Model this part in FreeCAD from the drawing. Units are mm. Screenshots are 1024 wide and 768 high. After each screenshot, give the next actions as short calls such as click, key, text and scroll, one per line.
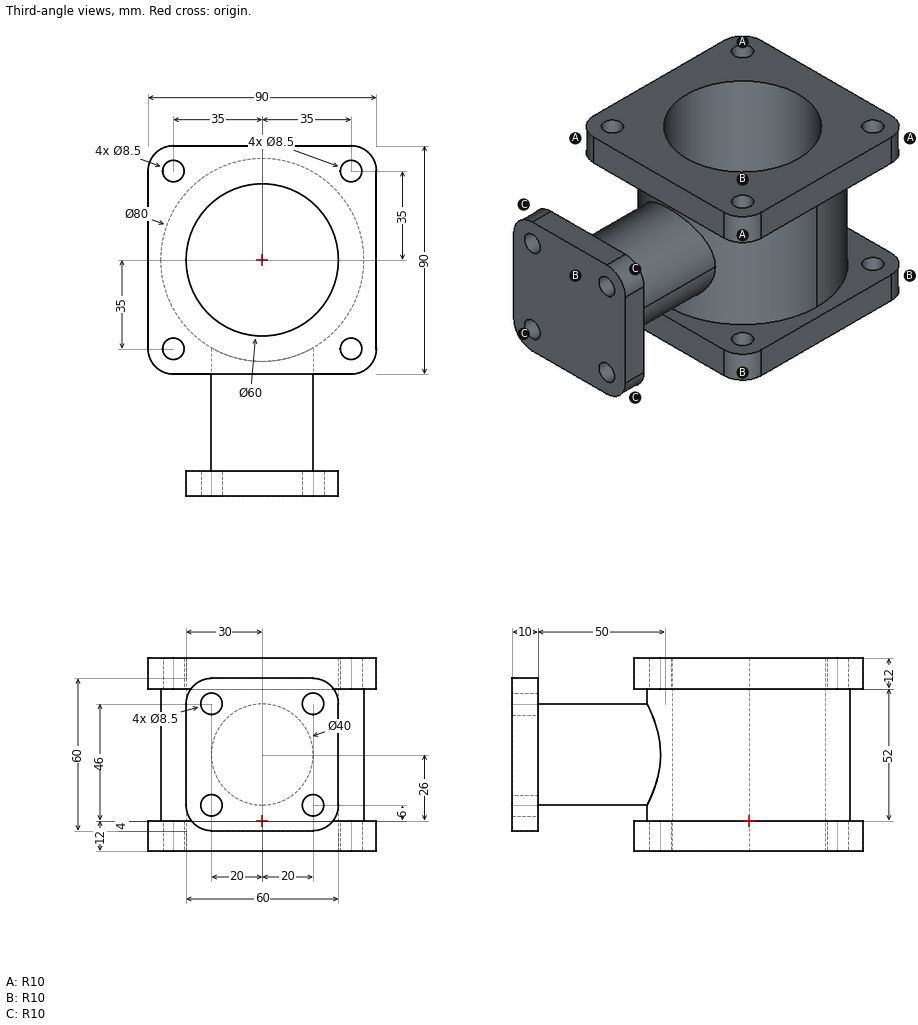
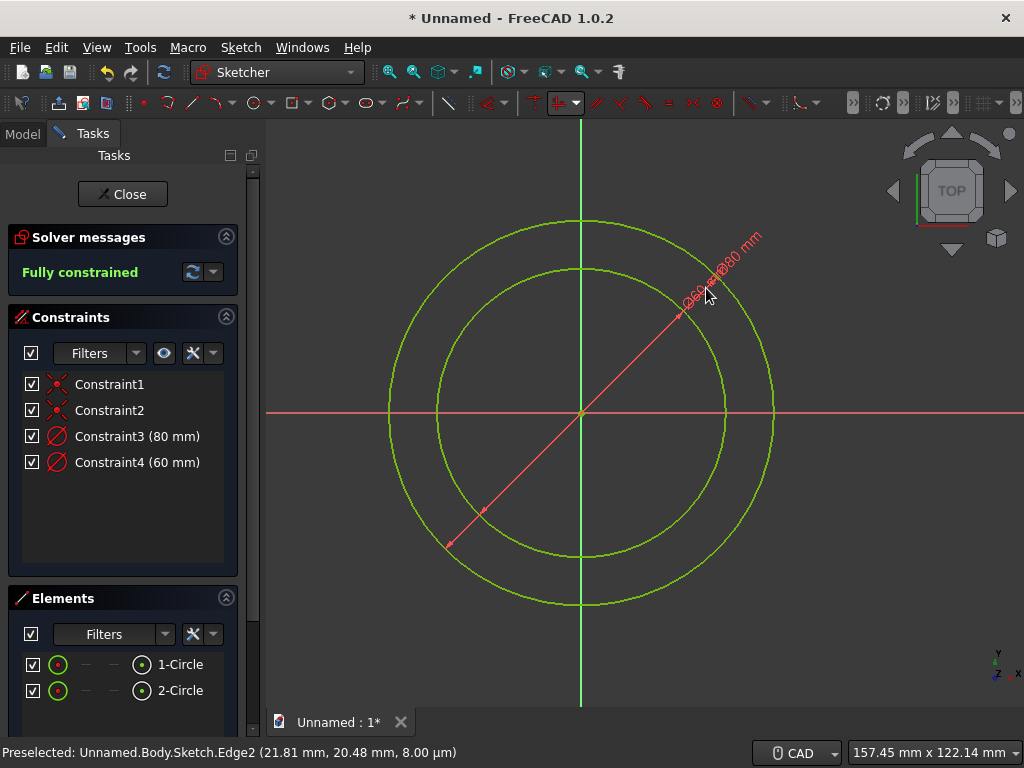
click(123, 194)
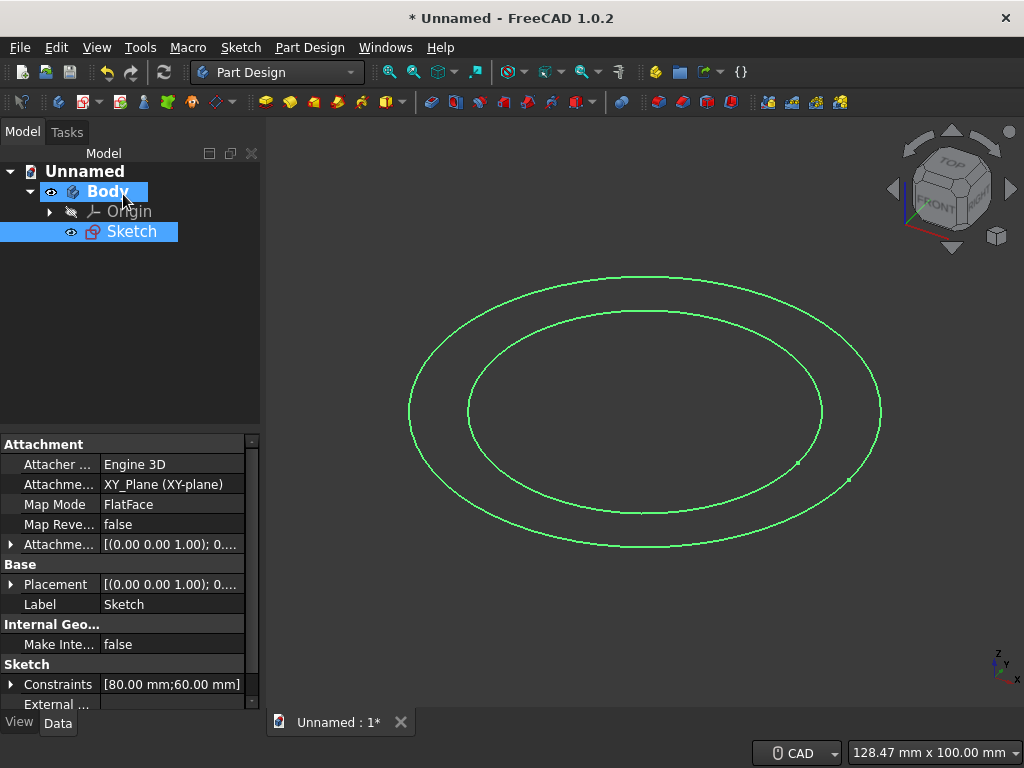
click(266, 102)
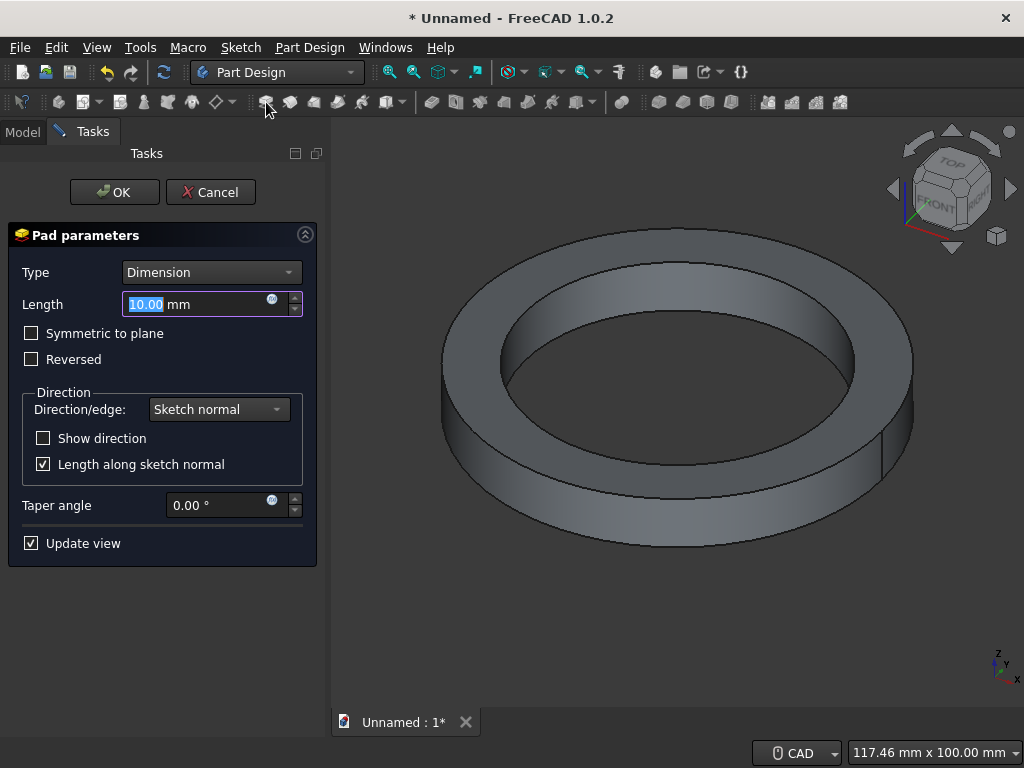
text(52)
key(Tab)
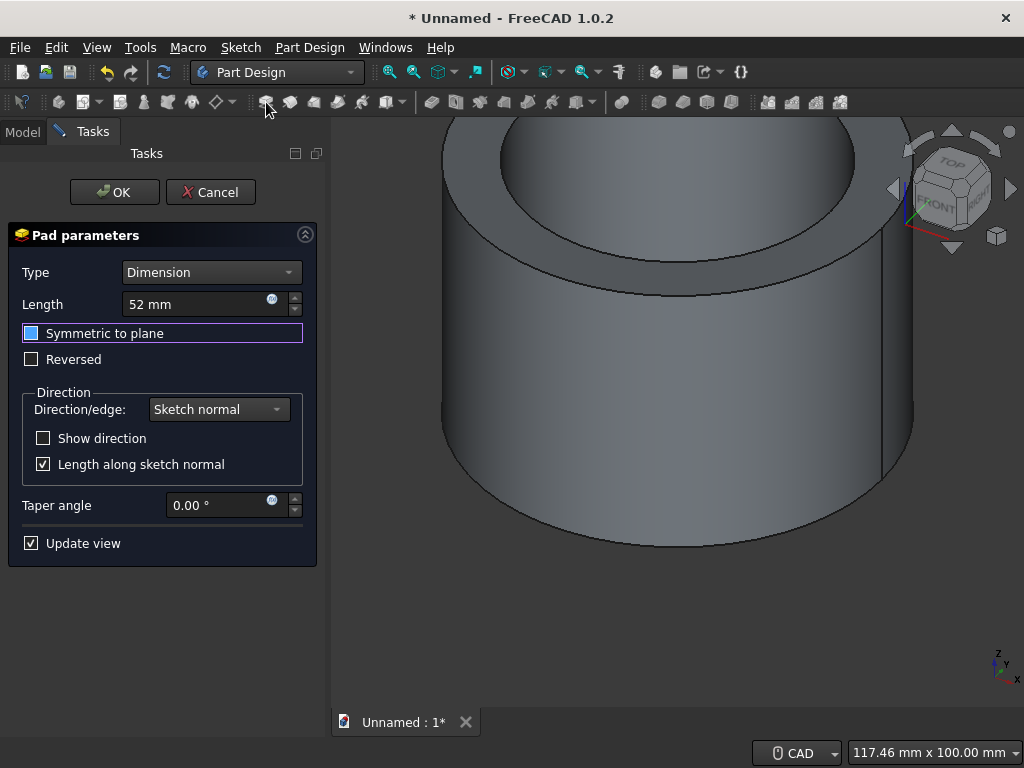
click(115, 192)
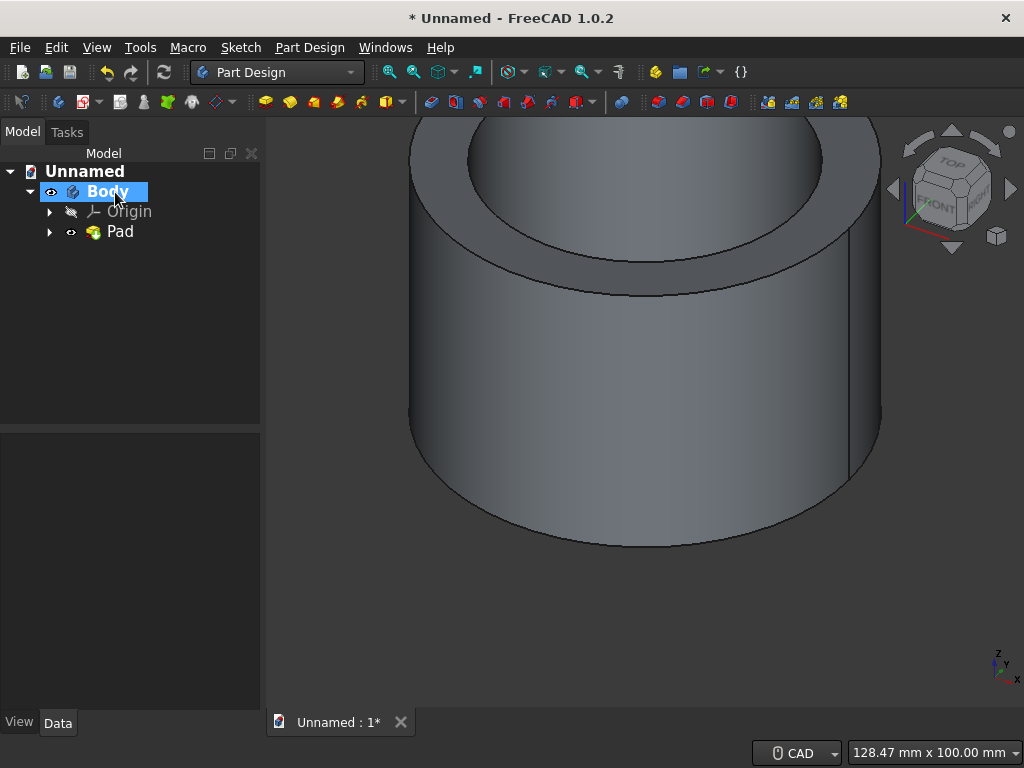
click(390, 72)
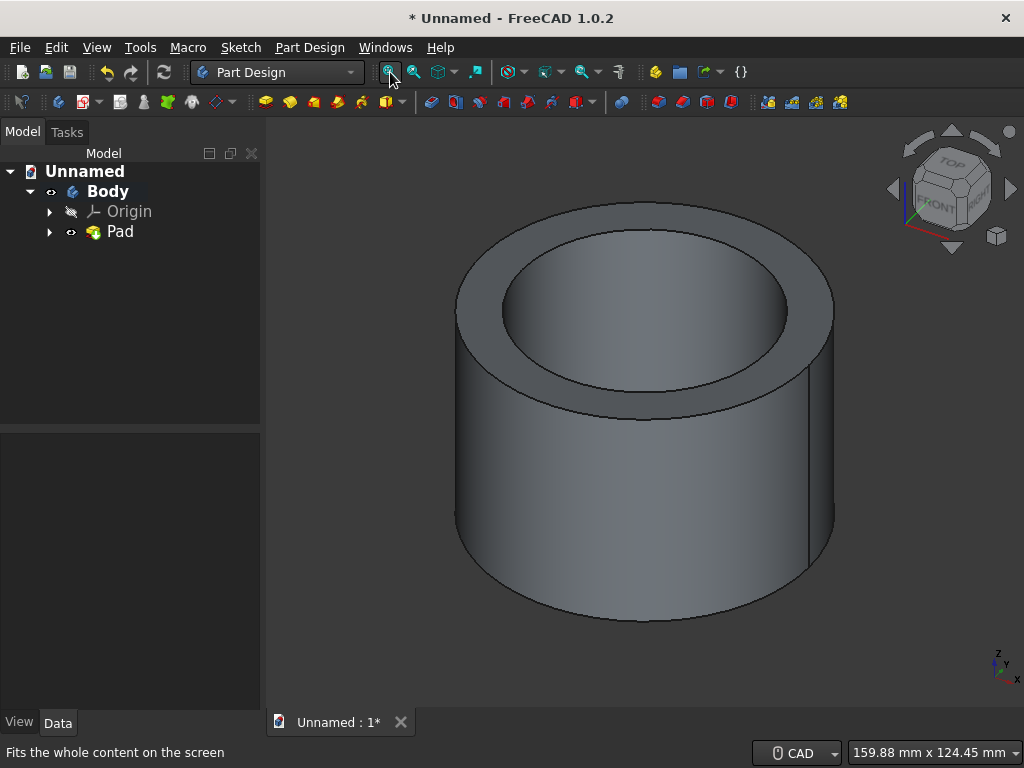
key(5)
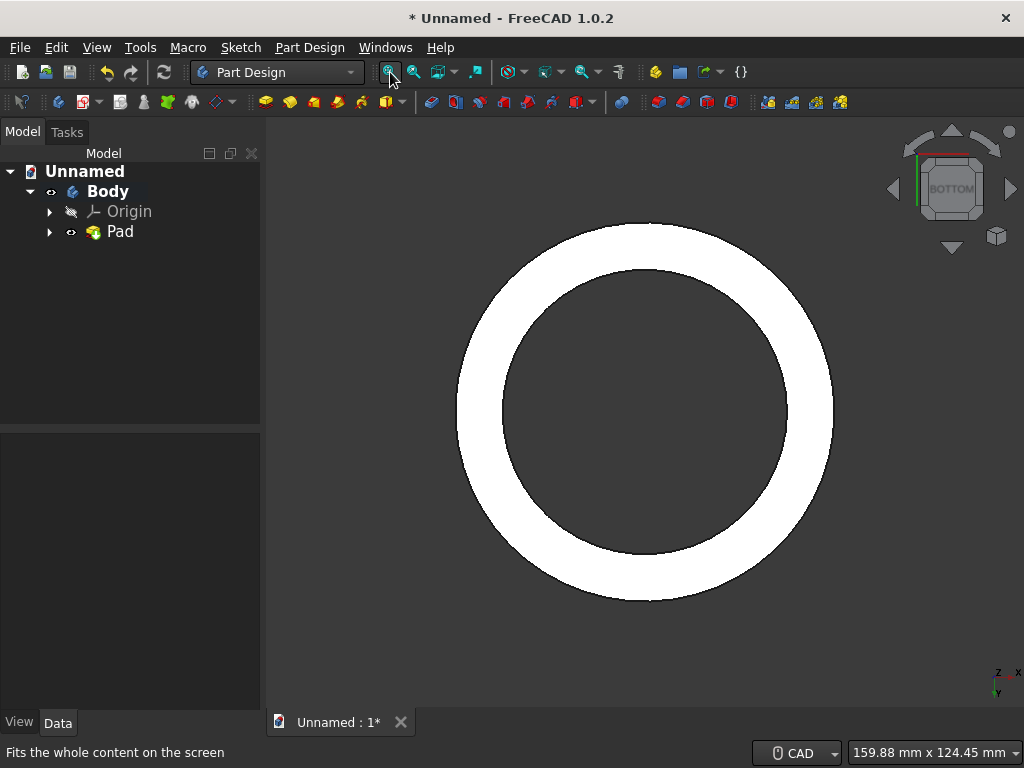
click(807, 411)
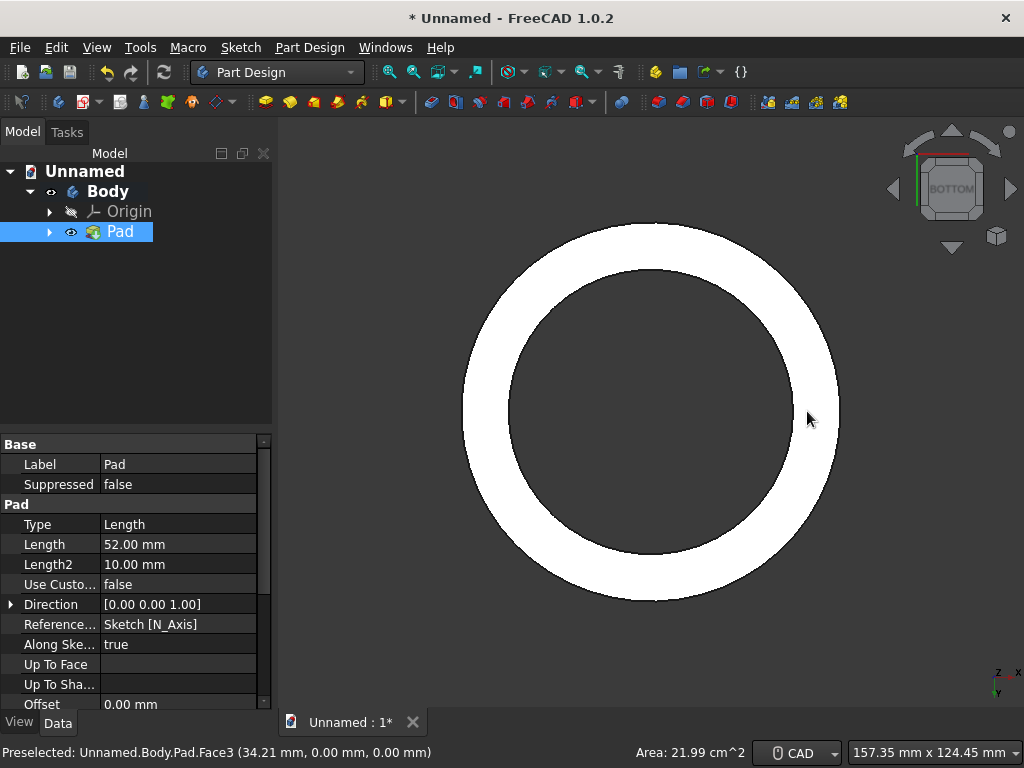
click(84, 102)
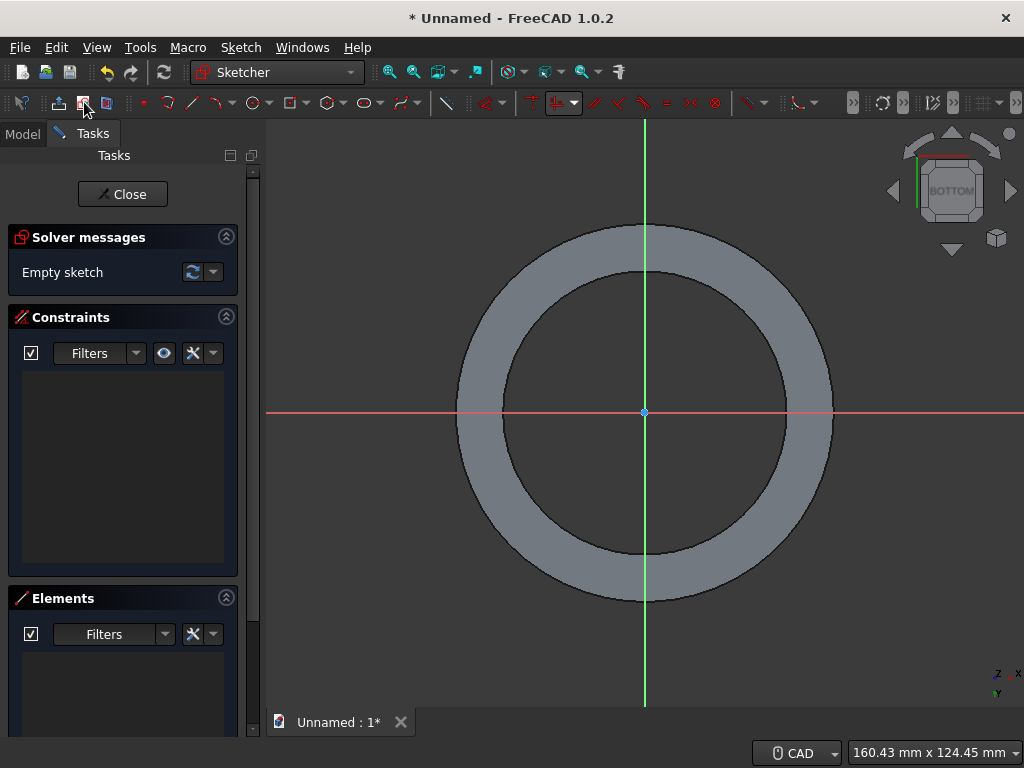
scroll(294, 413, down, 1)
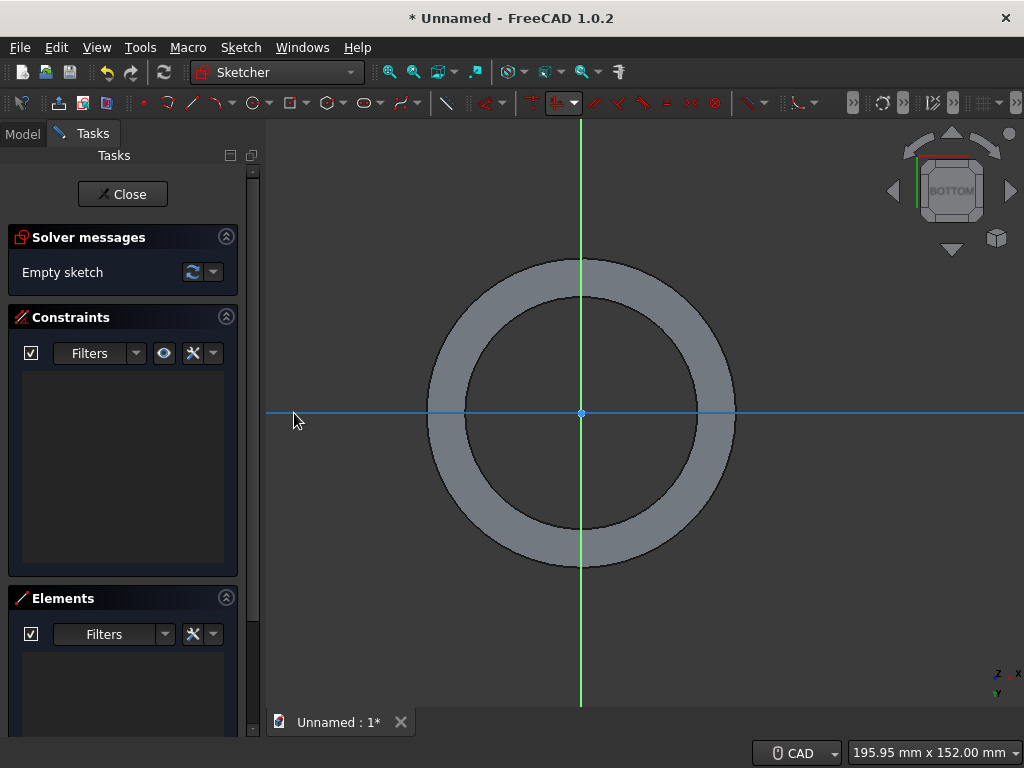
key(g)
key(v)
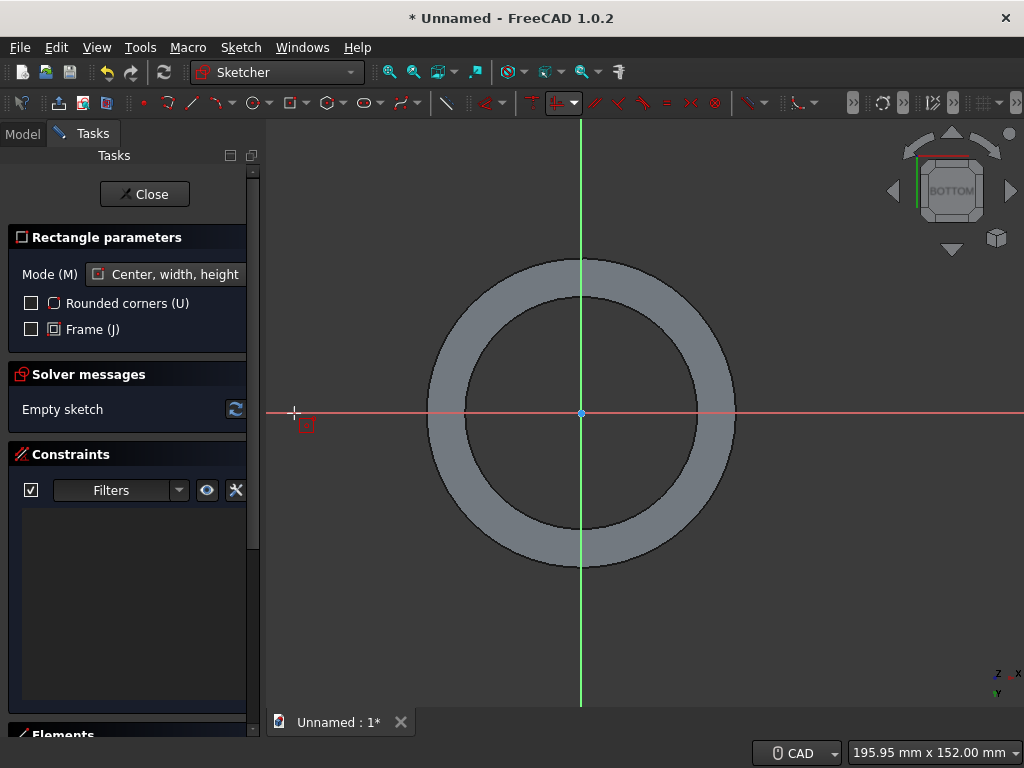
click(581, 413)
click(755, 239)
key(Escape)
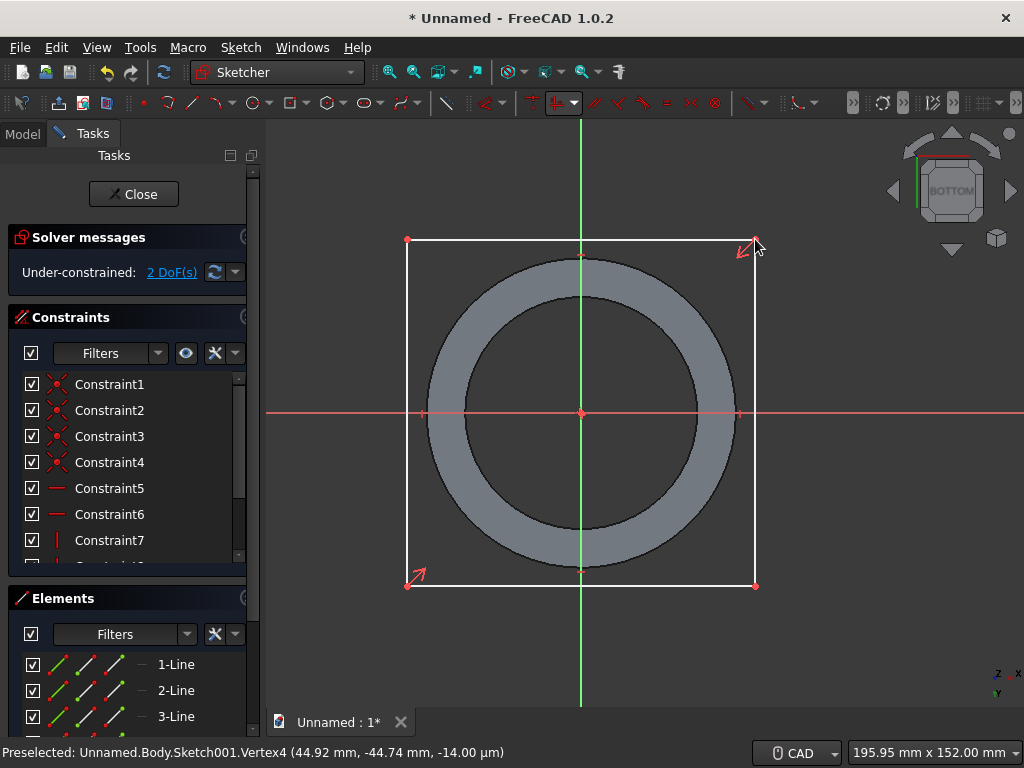
click(486, 104)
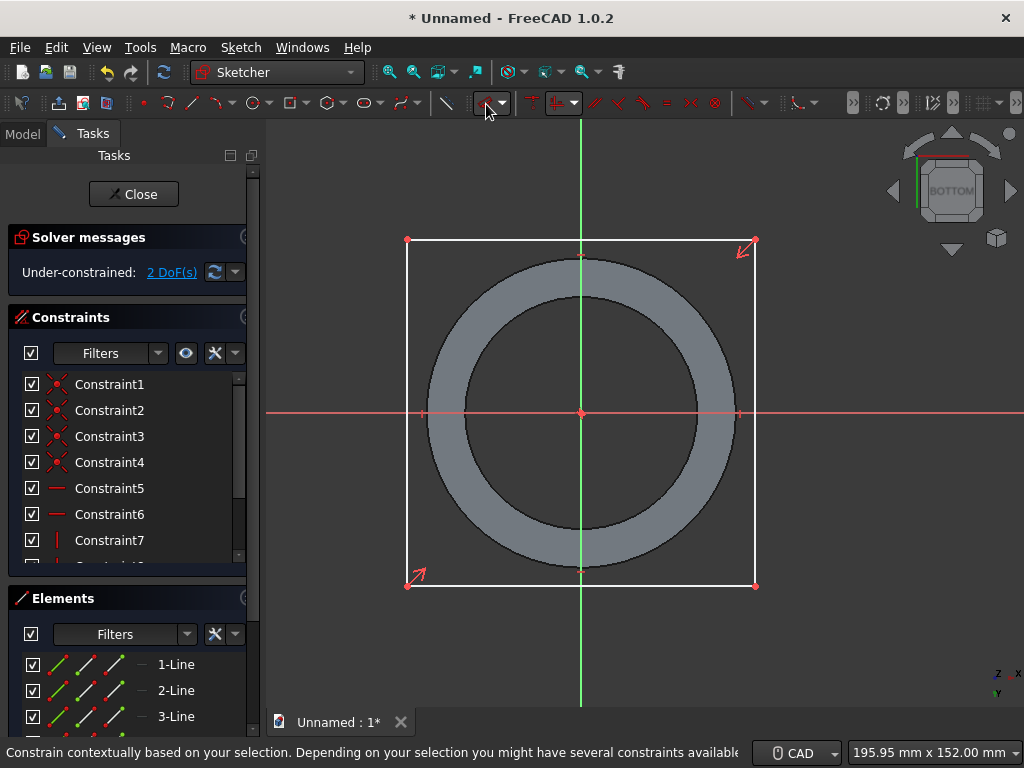
click(512, 586)
click(501, 620)